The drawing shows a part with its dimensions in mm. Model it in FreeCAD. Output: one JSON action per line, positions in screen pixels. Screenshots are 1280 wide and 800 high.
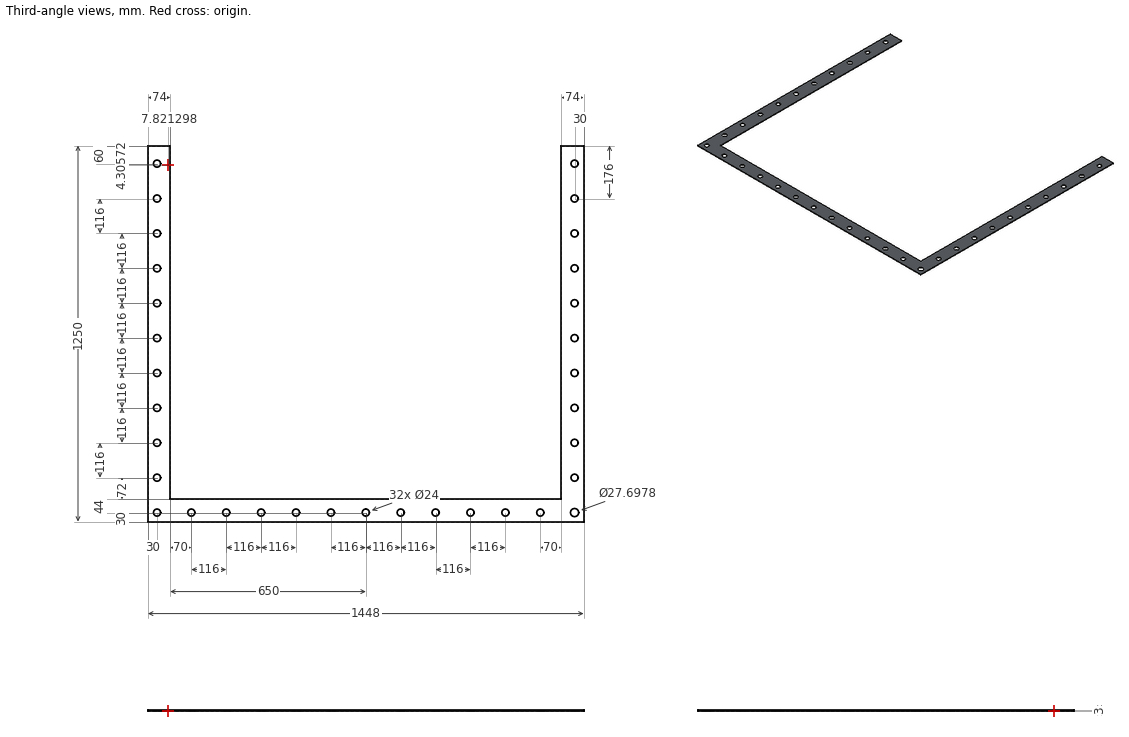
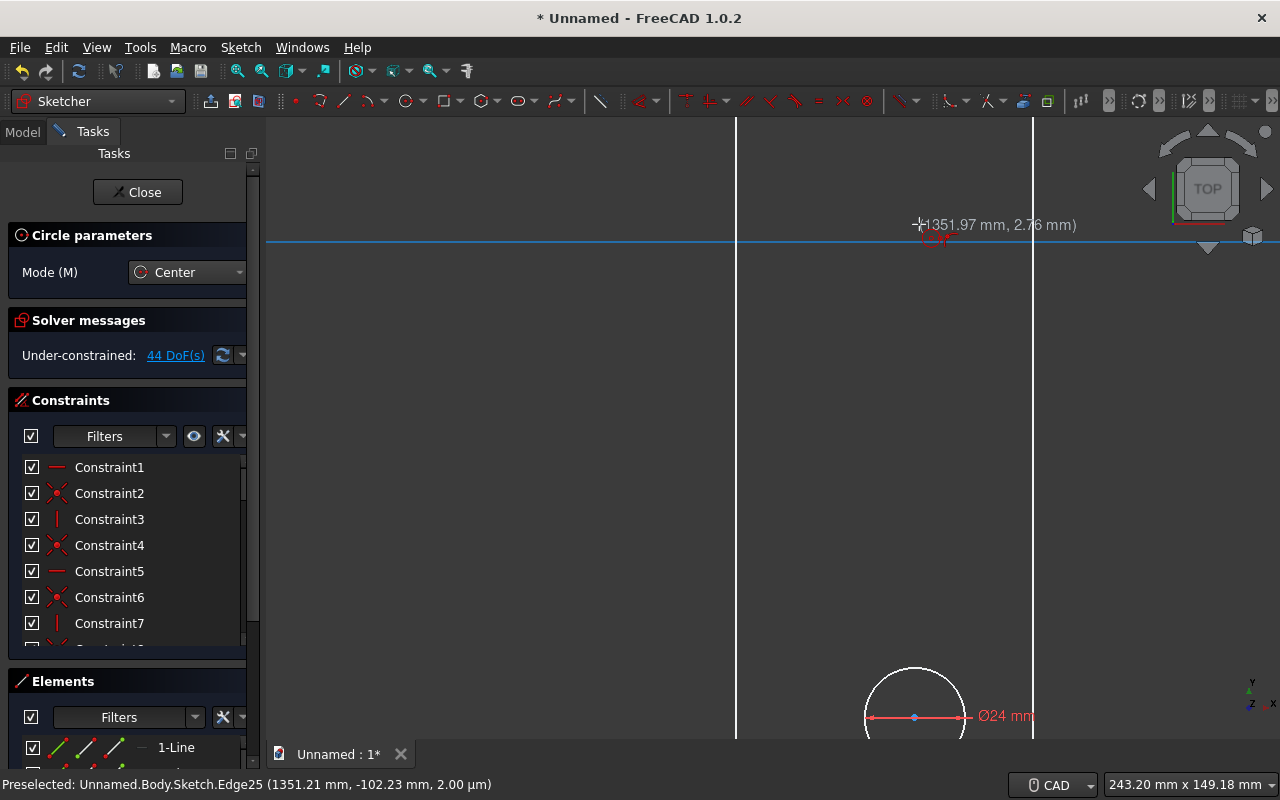
{"action": "left_click", "coordinate": [914, 224]}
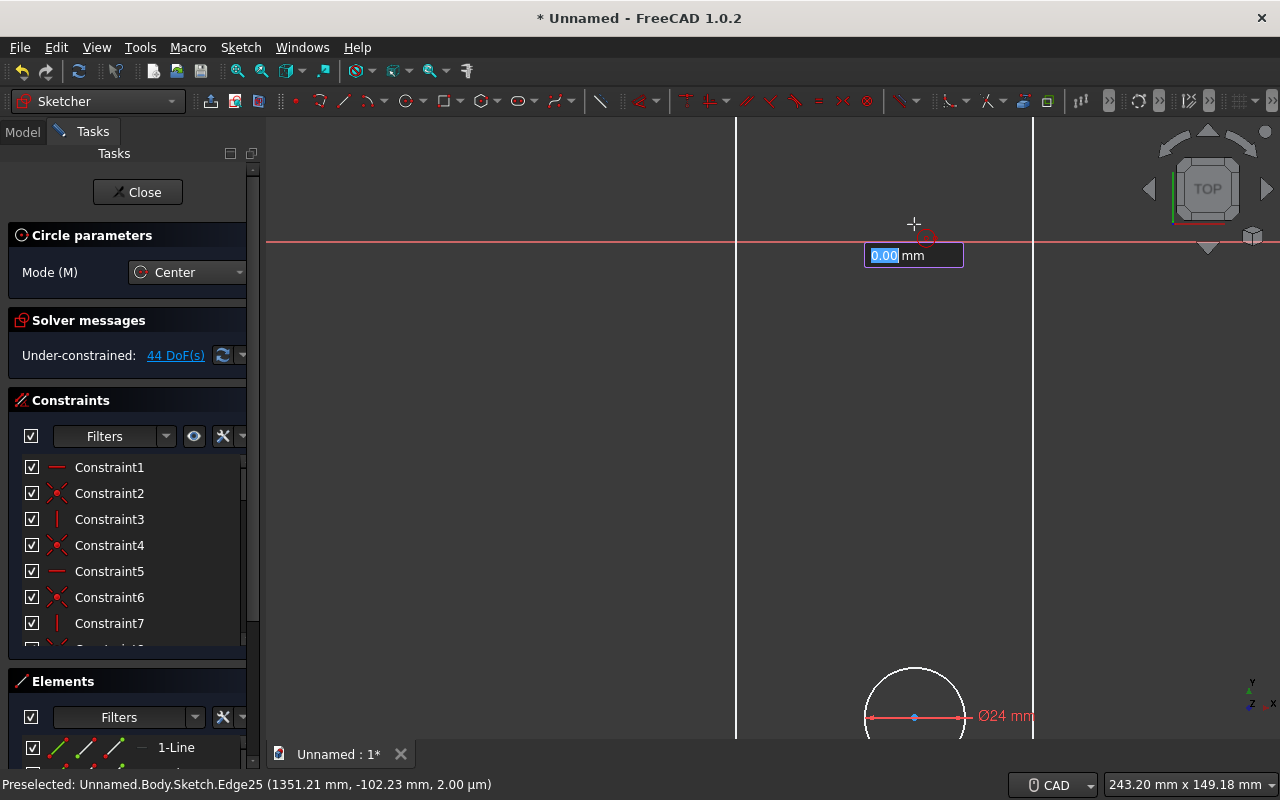
{"action": "scroll", "coordinate": [920, 255], "scroll_direction": "down", "scroll_amount": 13}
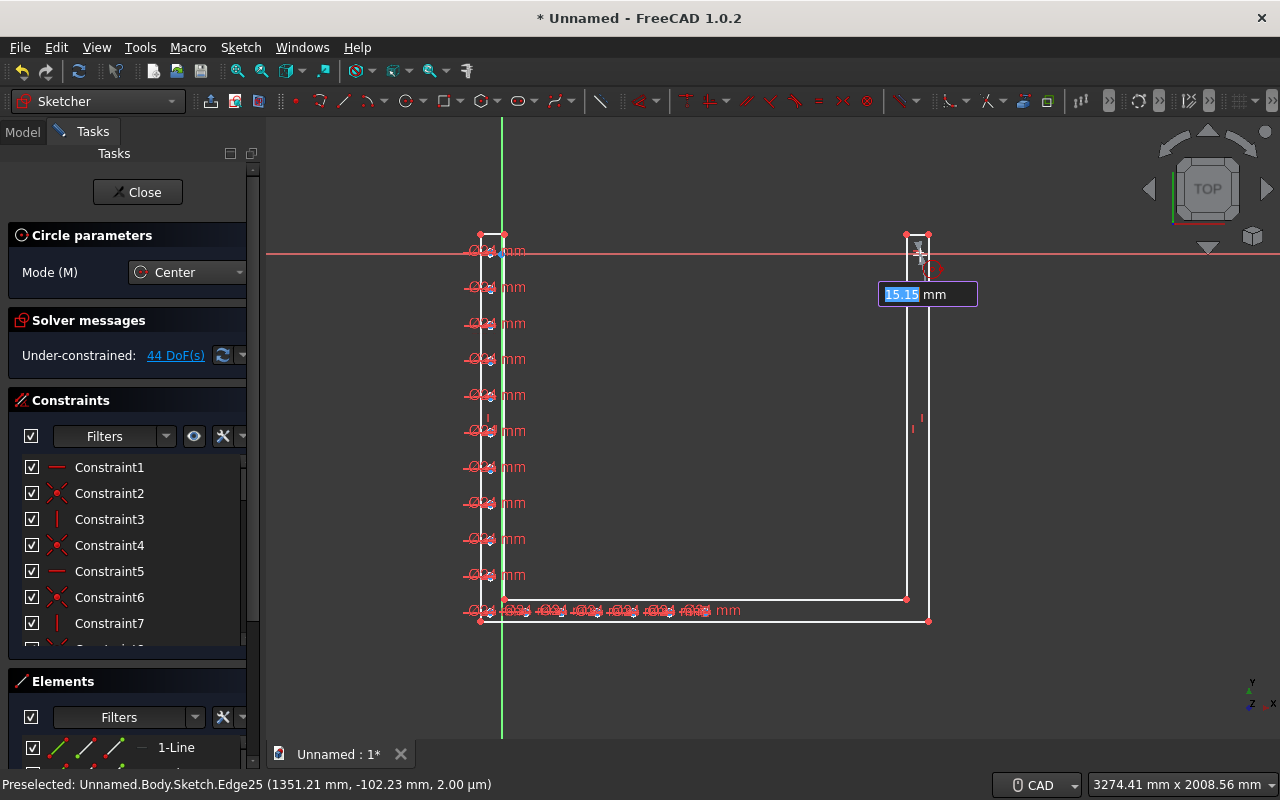
{"action": "scroll", "coordinate": [923, 250], "scroll_direction": "up", "scroll_amount": 7}
{"action": "mouse_move", "coordinate": [920, 250]}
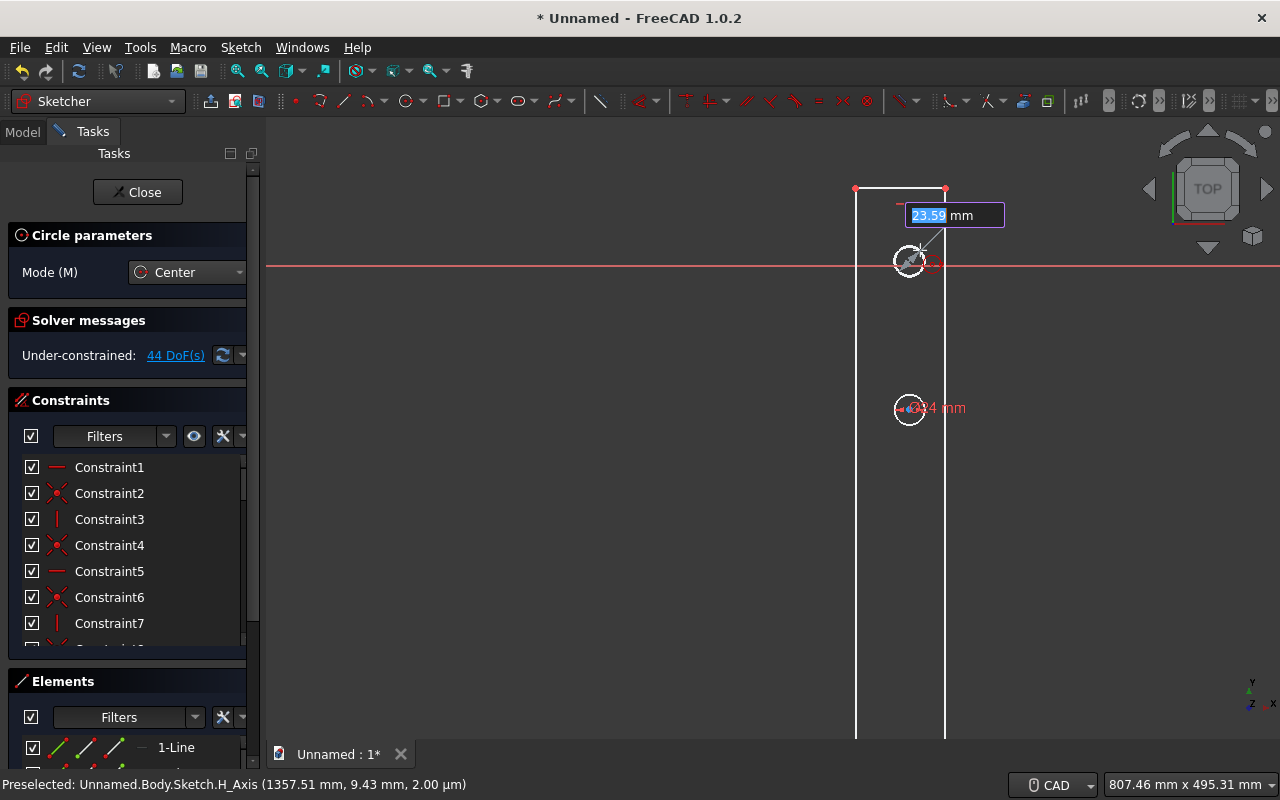
{"action": "type", "text": "24"}
{"action": "key", "text": "Return"}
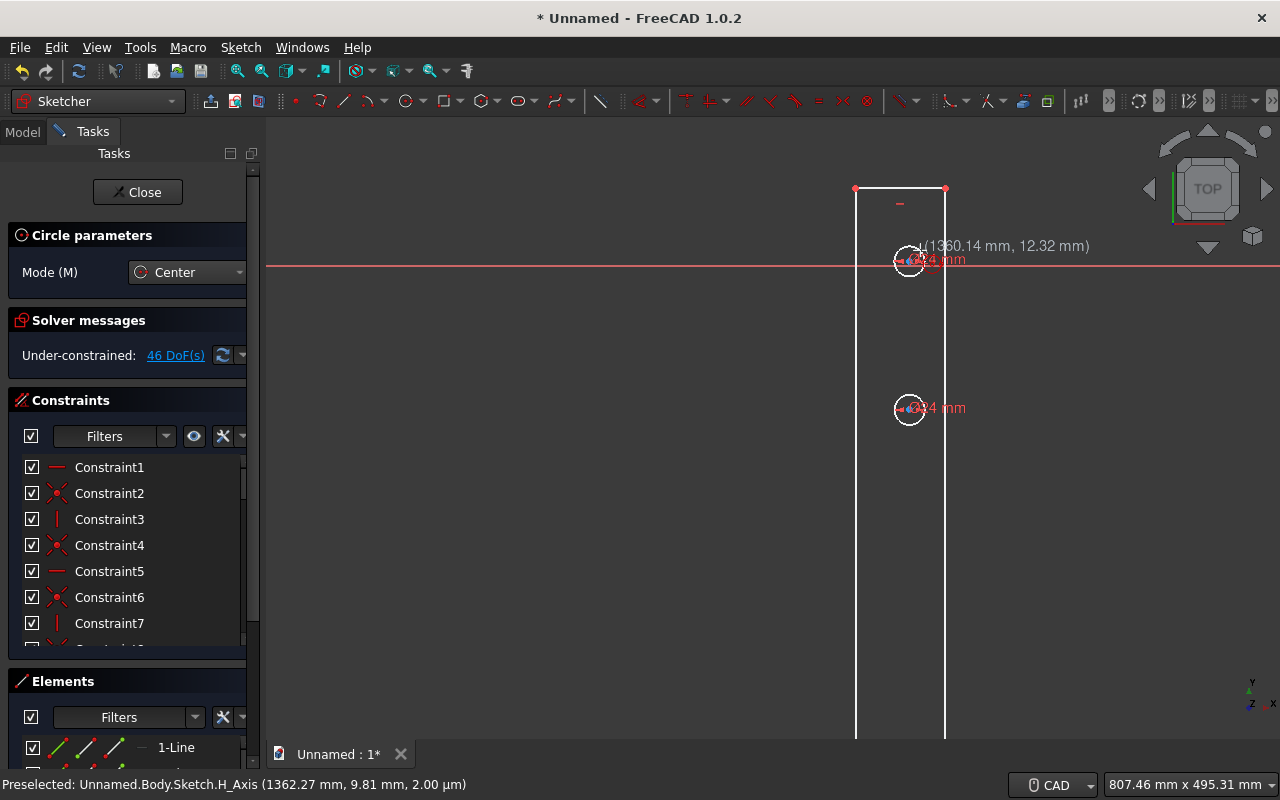
{"action": "scroll", "coordinate": [923, 250], "scroll_direction": "down", "scroll_amount": 7}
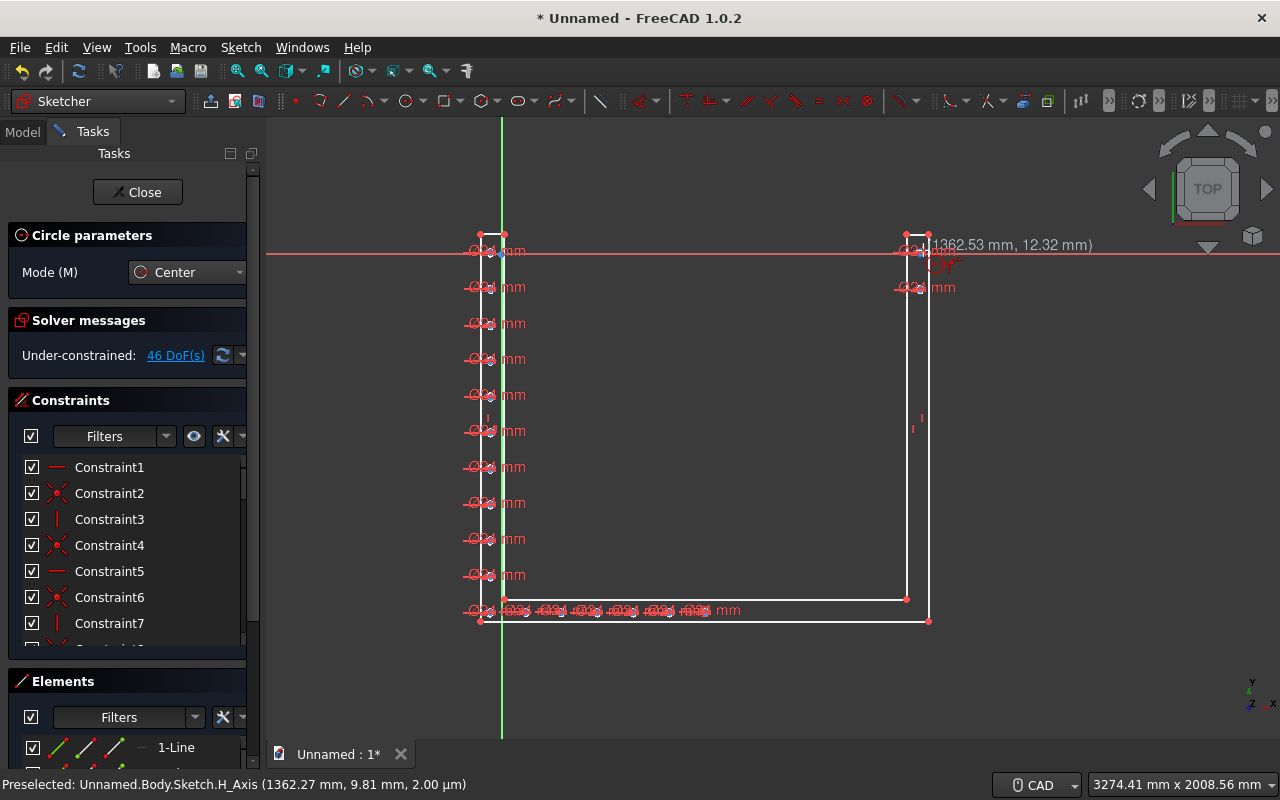
{"action": "scroll", "coordinate": [741, 612], "scroll_direction": "up", "scroll_amount": 10}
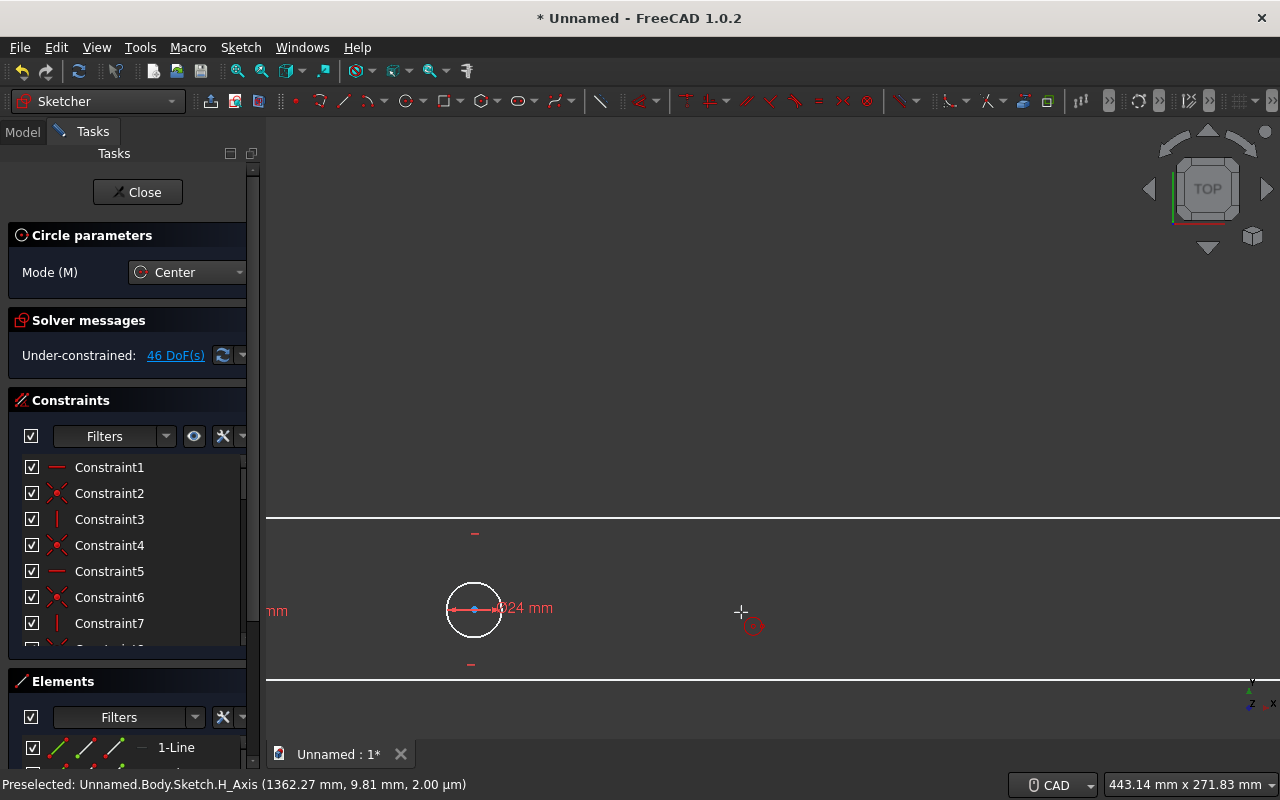
{"action": "scroll", "coordinate": [741, 613], "scroll_direction": "down", "scroll_amount": 10}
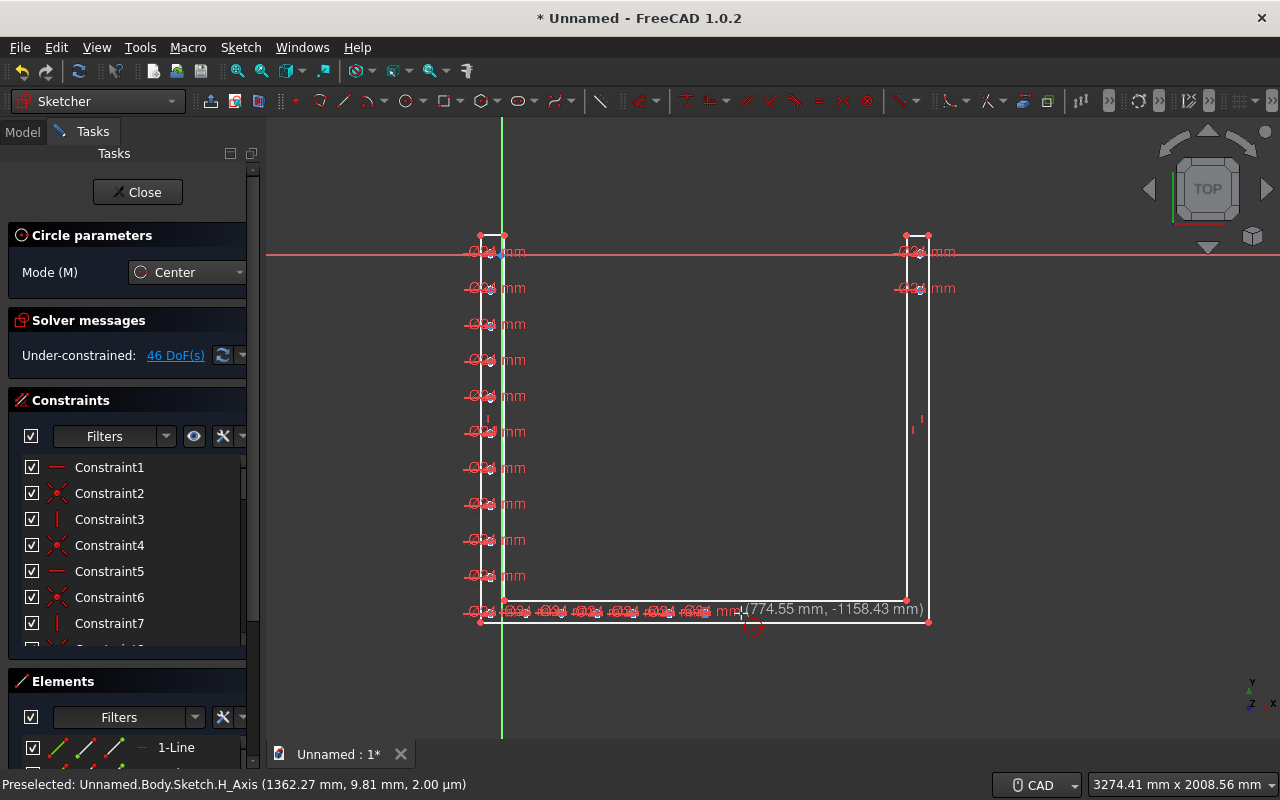
{"action": "scroll", "coordinate": [741, 613], "scroll_direction": "up", "scroll_amount": 3}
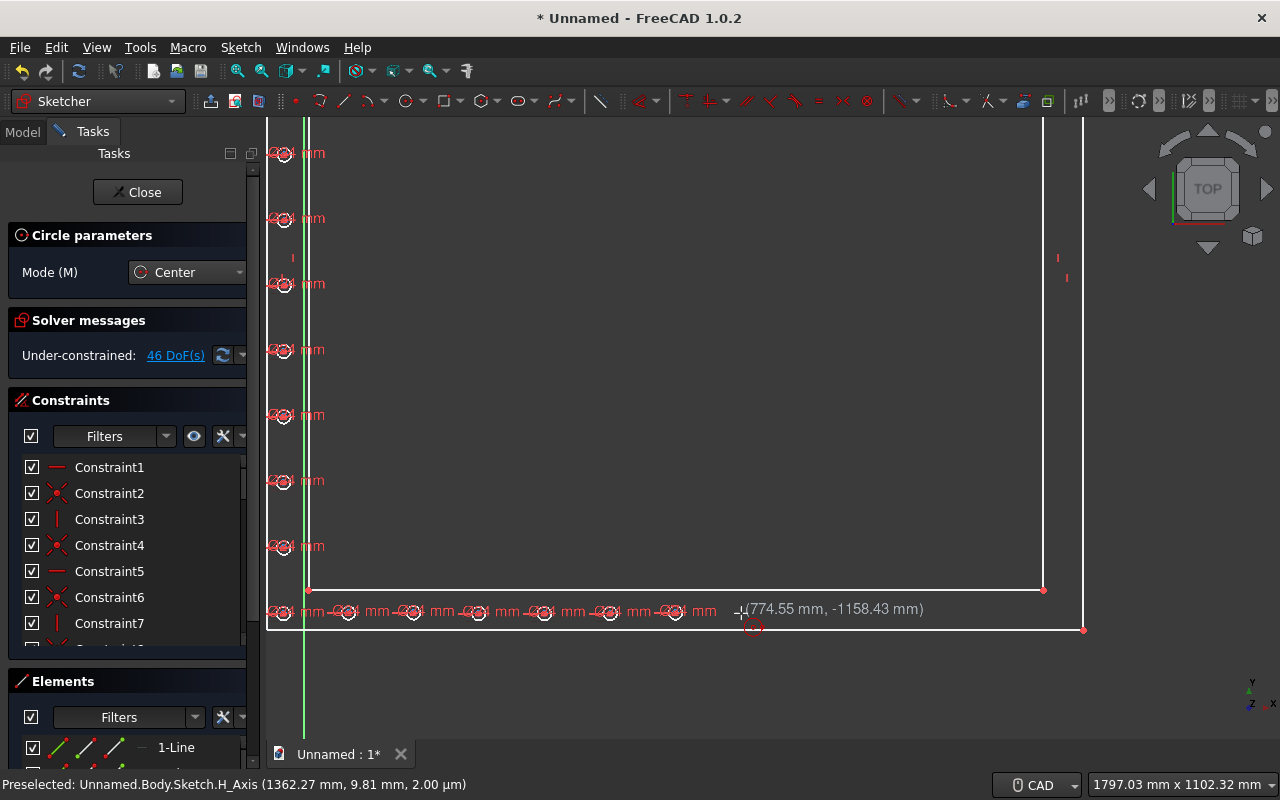
{"action": "left_click", "coordinate": [741, 612]}
{"action": "mouse_move", "coordinate": [746, 608]}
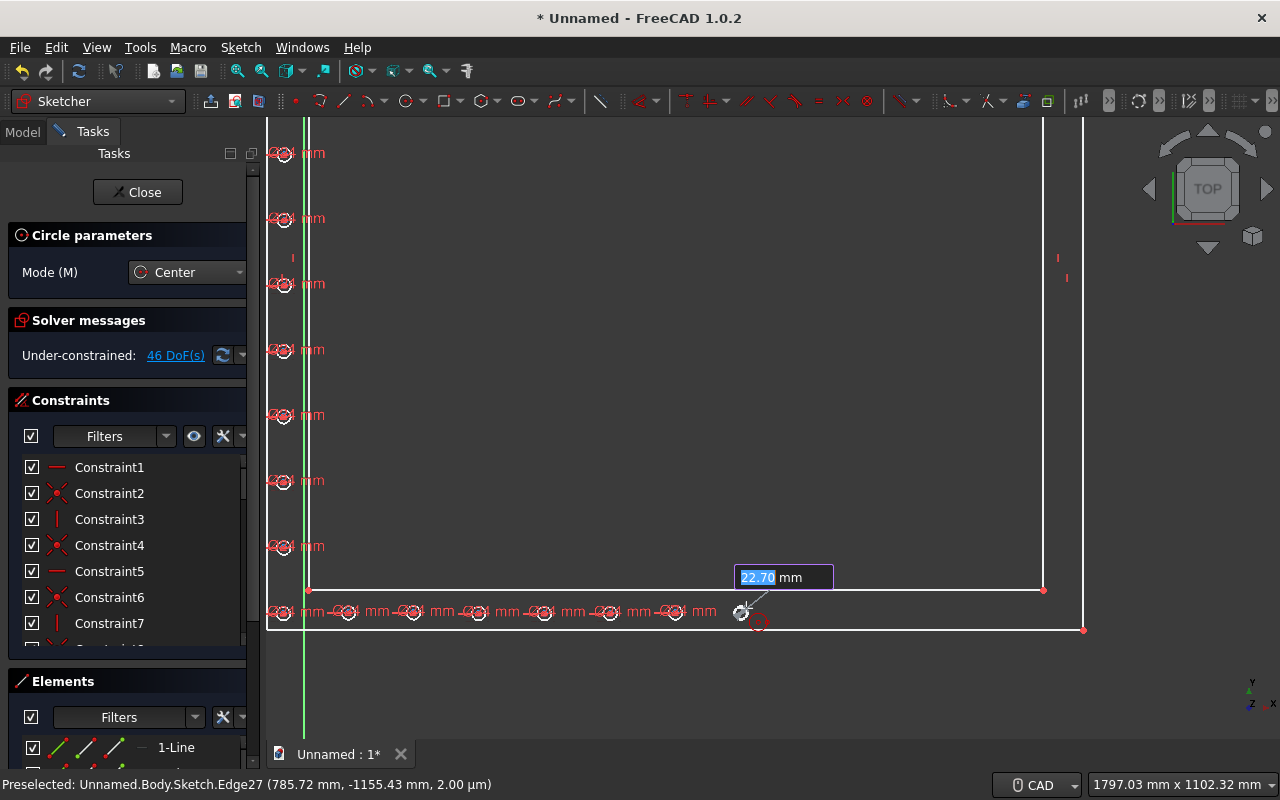
{"action": "type", "text": "24"}
{"action": "key", "text": "Return"}